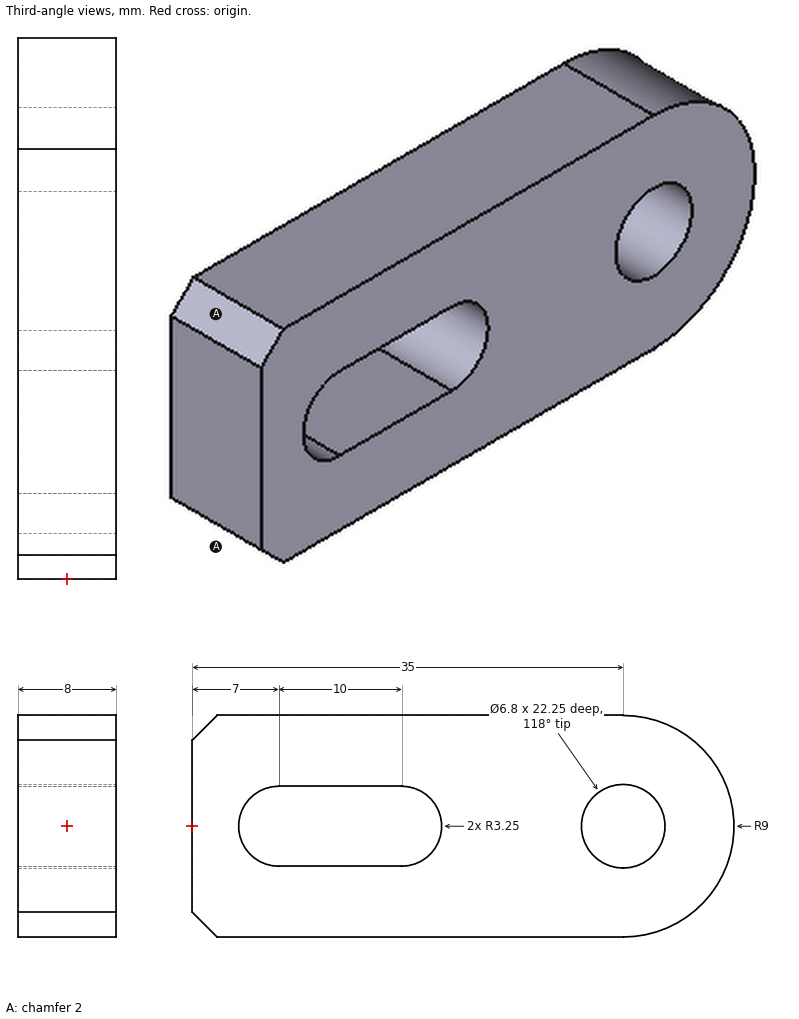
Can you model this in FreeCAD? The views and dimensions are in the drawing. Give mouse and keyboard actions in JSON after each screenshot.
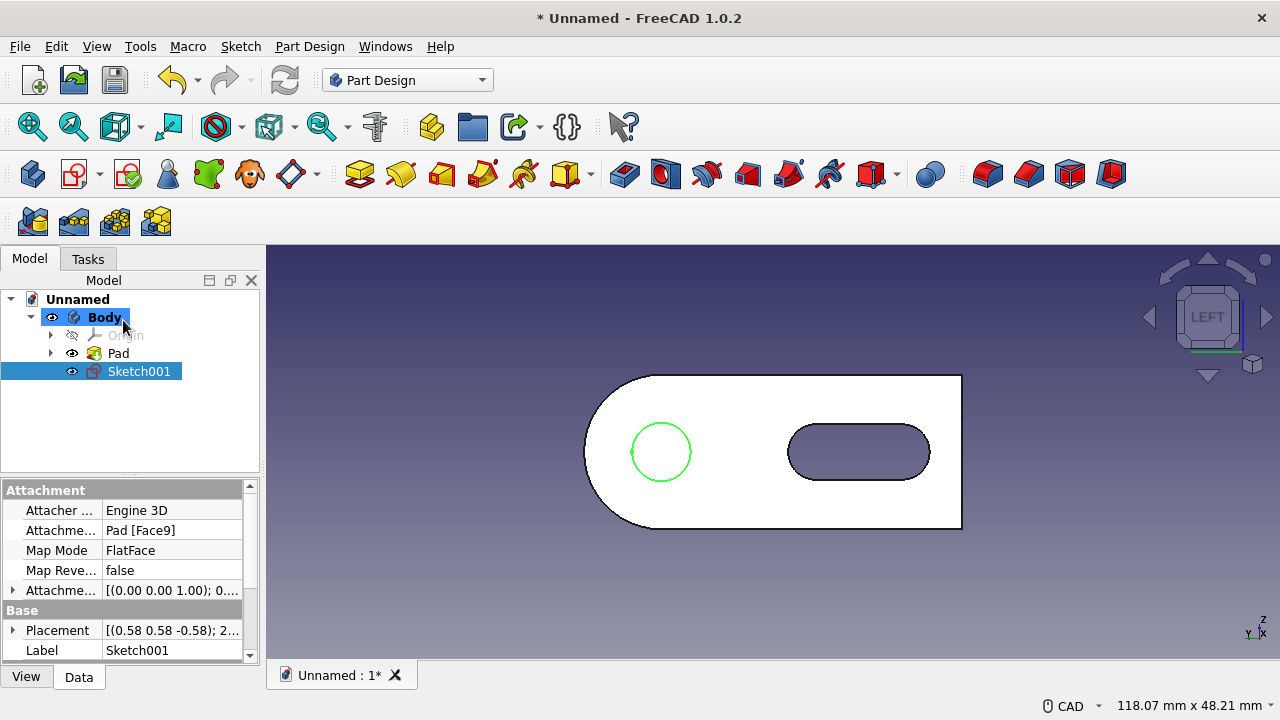
{"action": "left_click", "coordinate": [666, 174]}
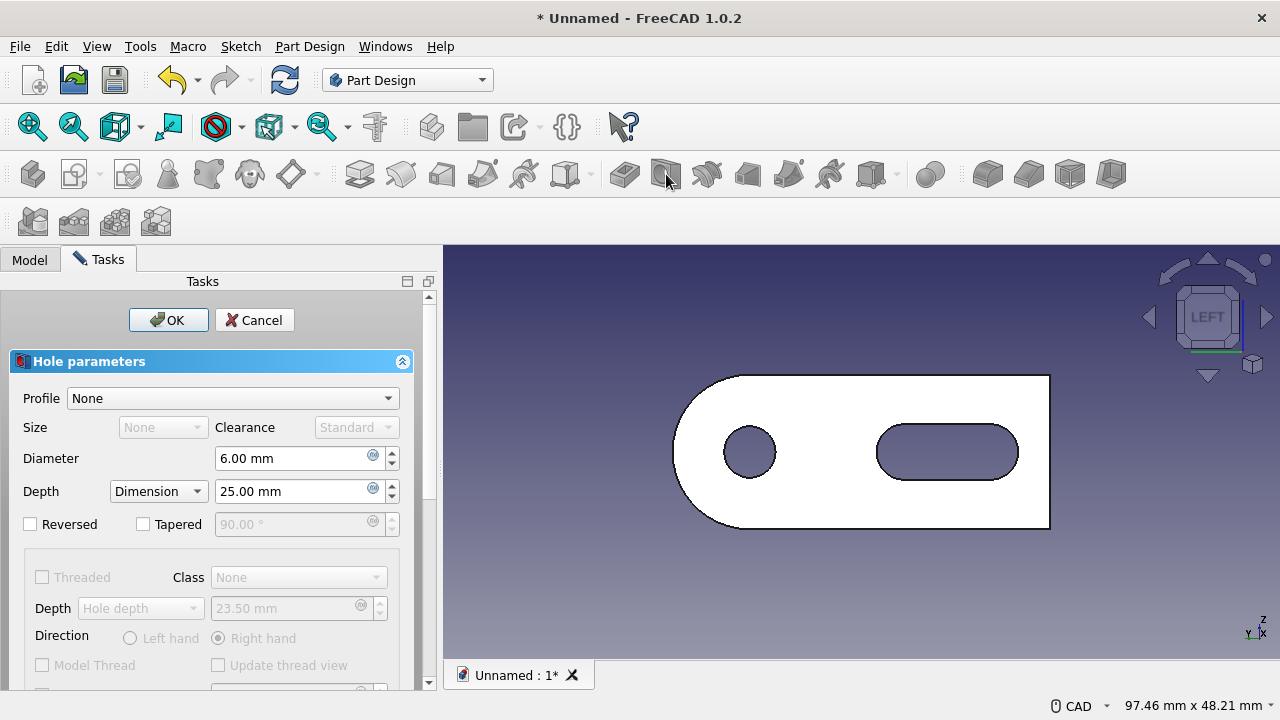
{"action": "triple_click", "coordinate": [300, 458]}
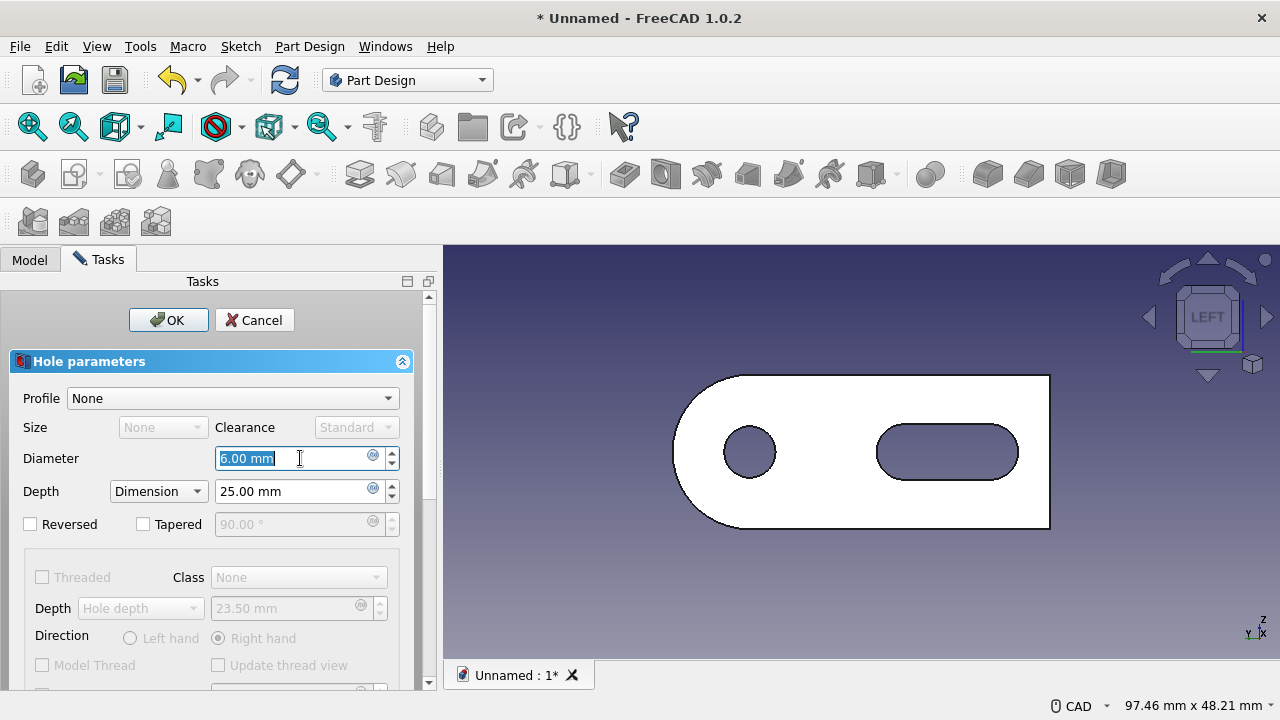
{"action": "type", "text": "6.8"}
{"action": "key", "text": "Tab"}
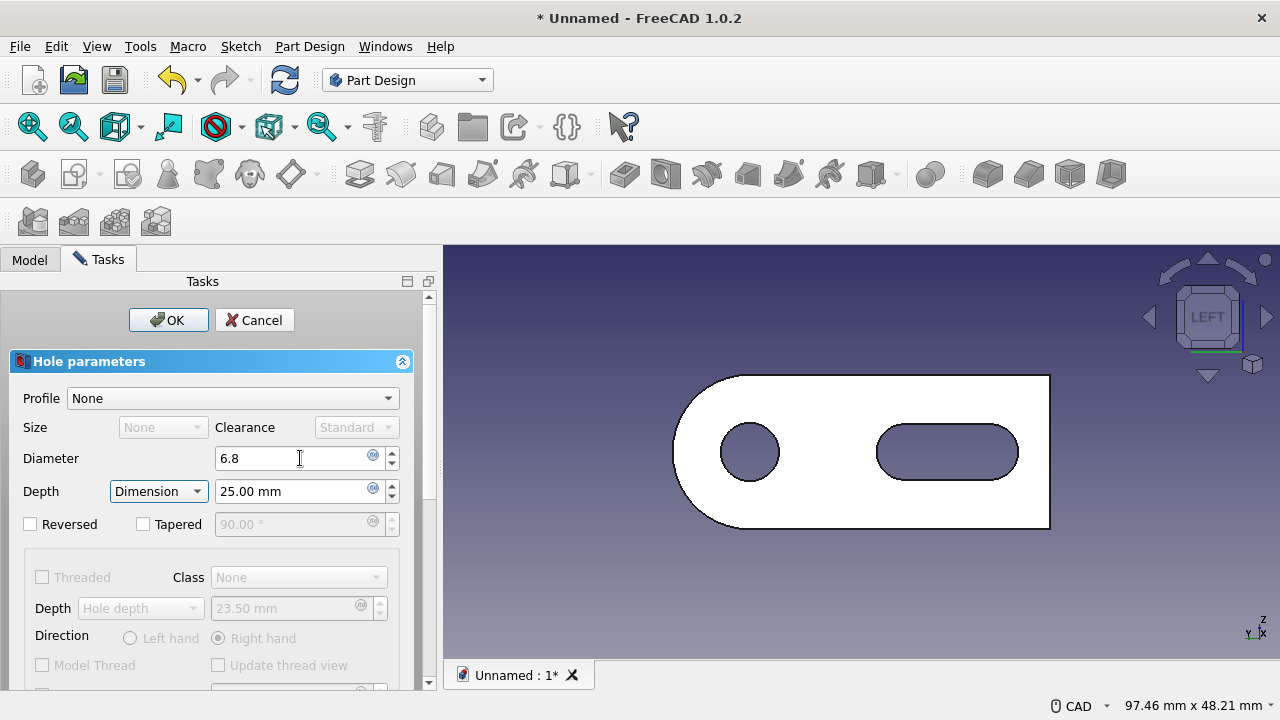
{"action": "triple_click", "coordinate": [300, 492]}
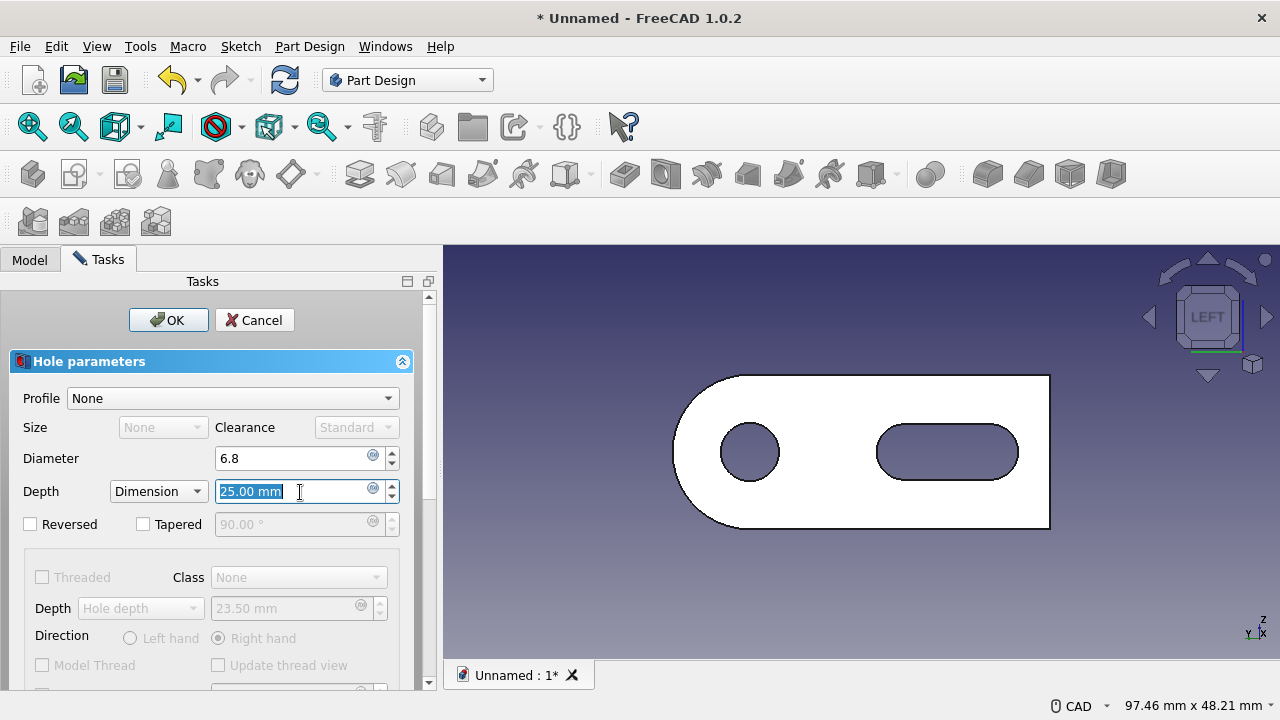
{"action": "type", "text": "22.25"}
{"action": "key", "text": "Tab"}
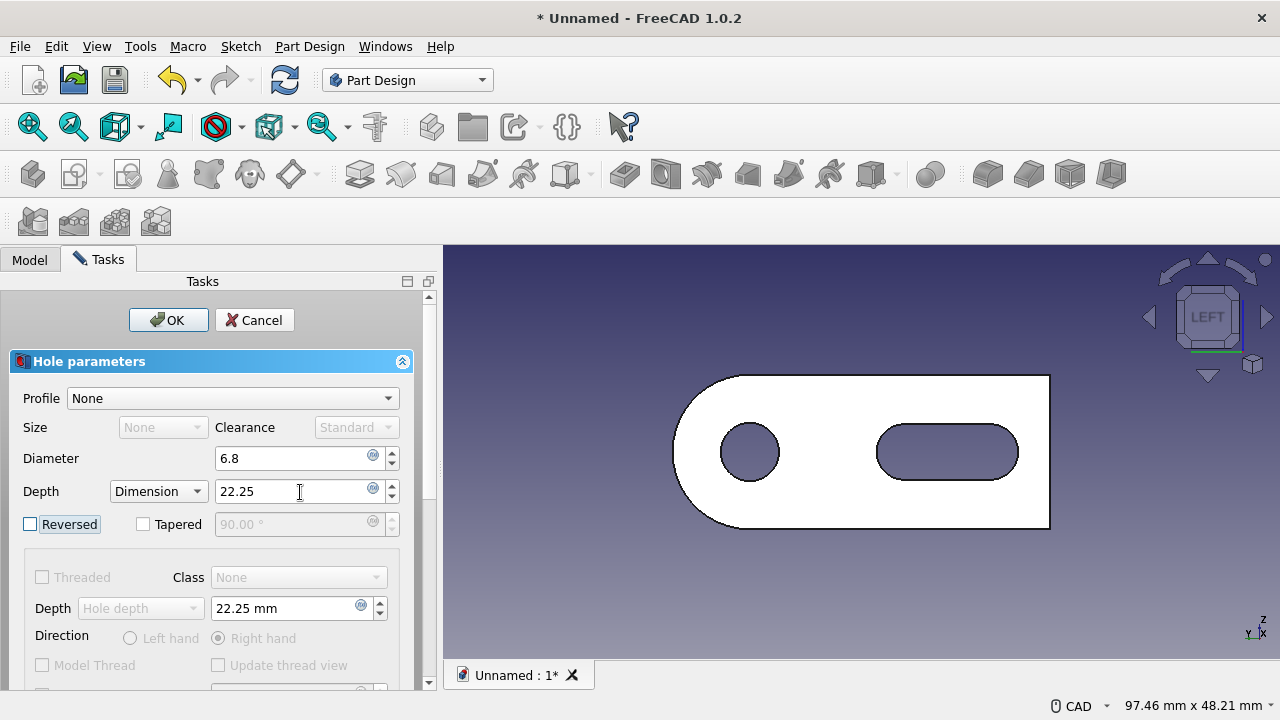
{"action": "left_click", "coordinate": [169, 320]}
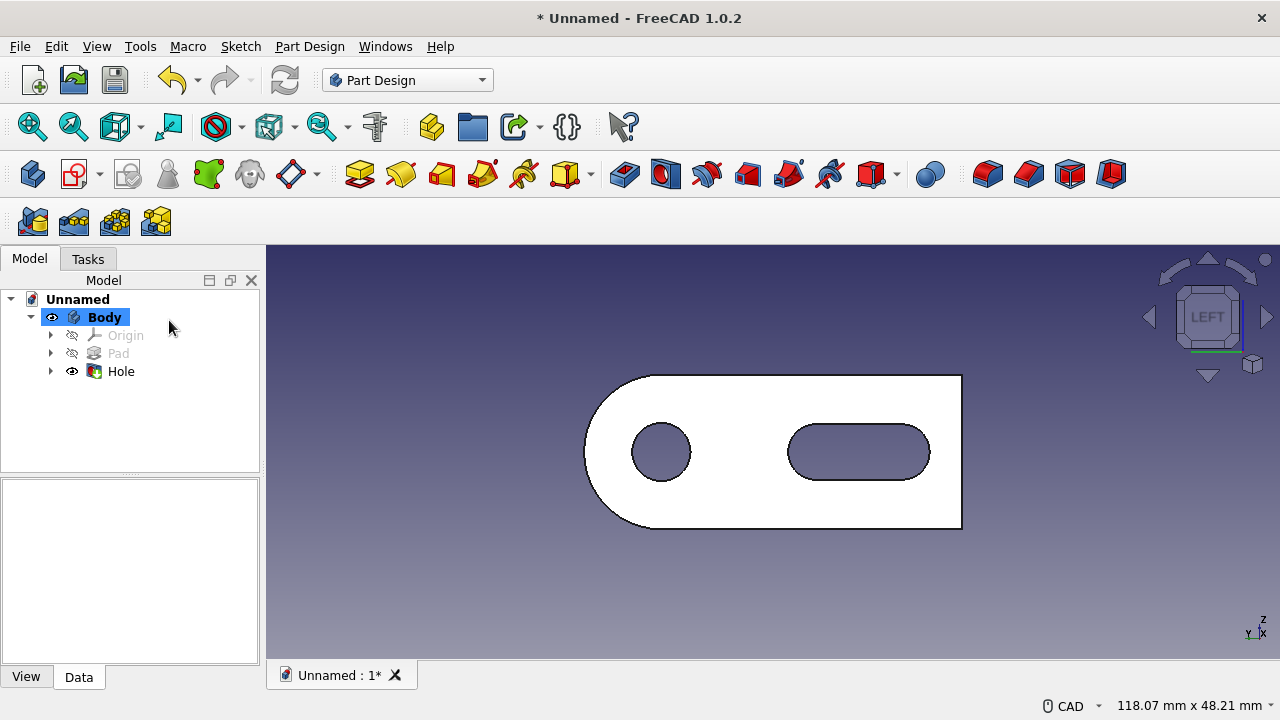
{"action": "key", "text": "v f"}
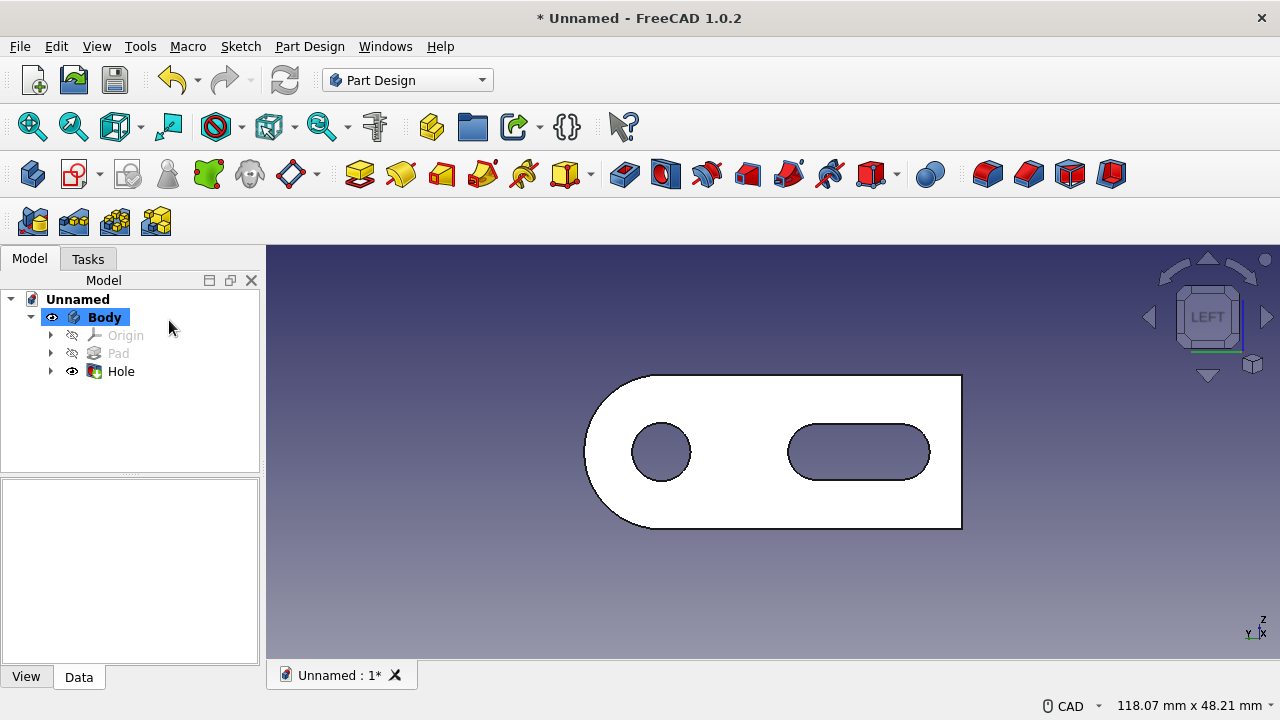
{"action": "key", "text": "0"}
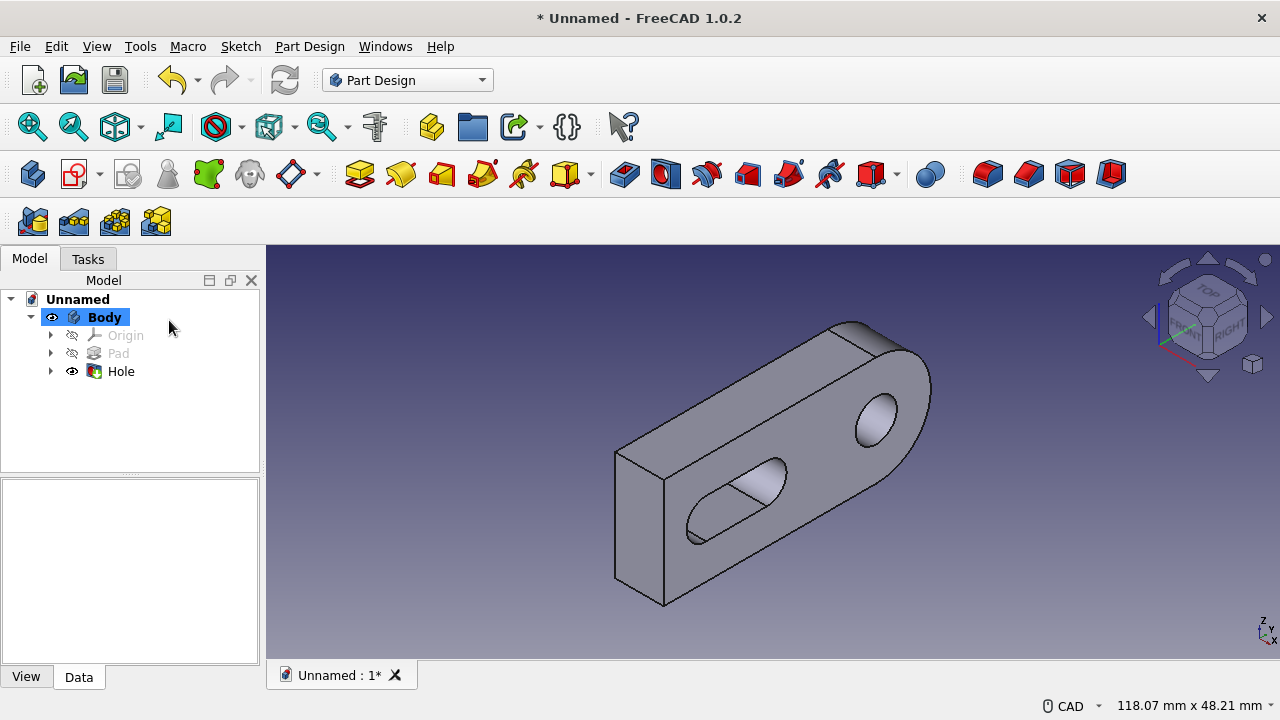
{"action": "left_click", "coordinate": [639, 465]}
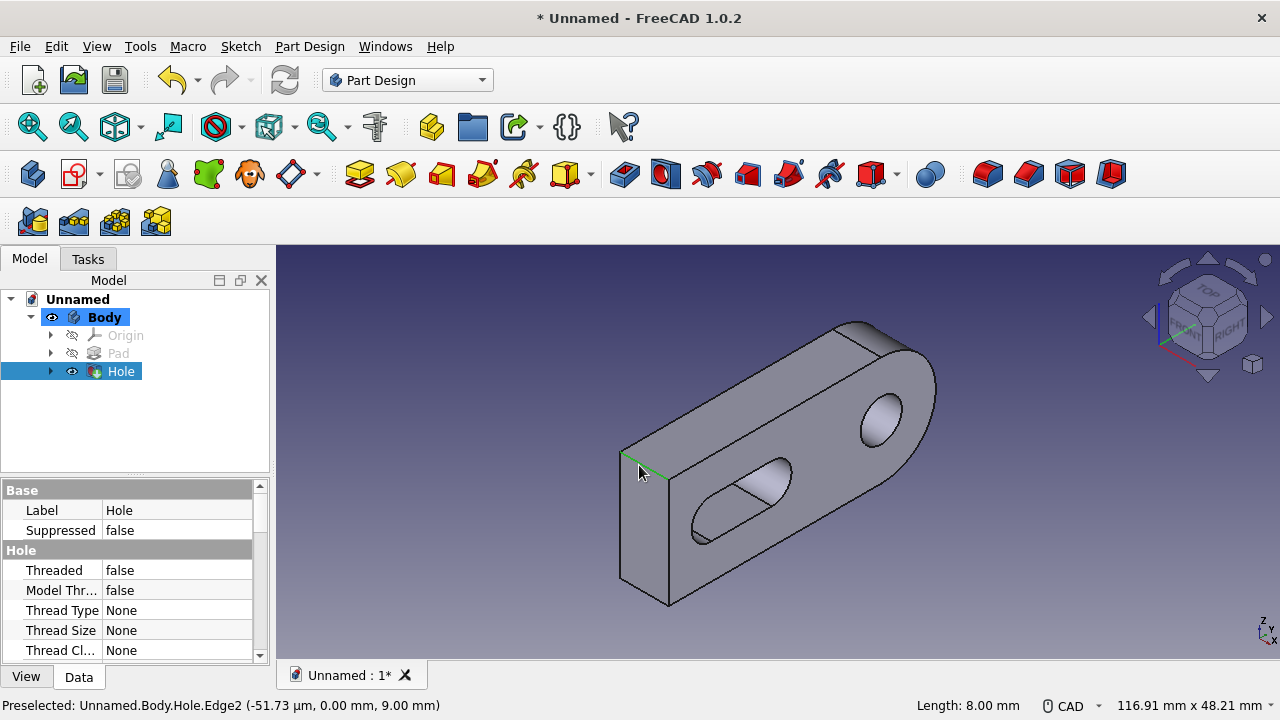
{"action": "key", "text": "2"}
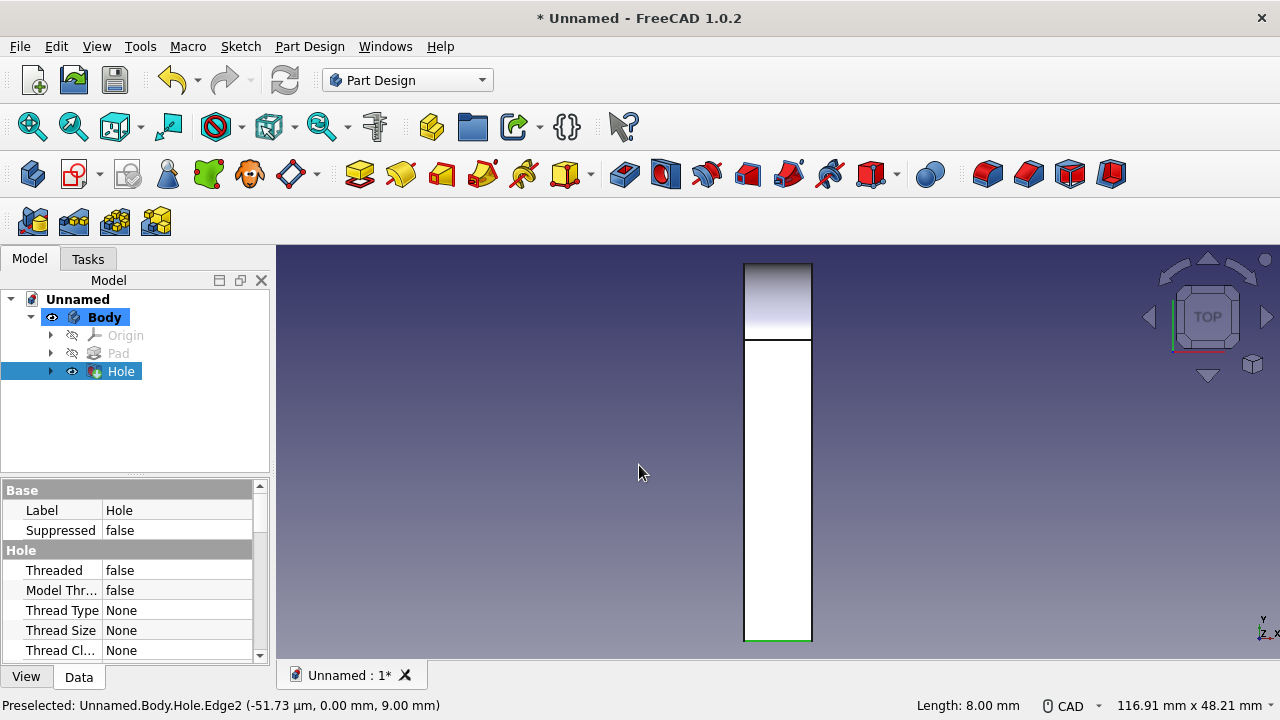
{"action": "key", "text": "1"}